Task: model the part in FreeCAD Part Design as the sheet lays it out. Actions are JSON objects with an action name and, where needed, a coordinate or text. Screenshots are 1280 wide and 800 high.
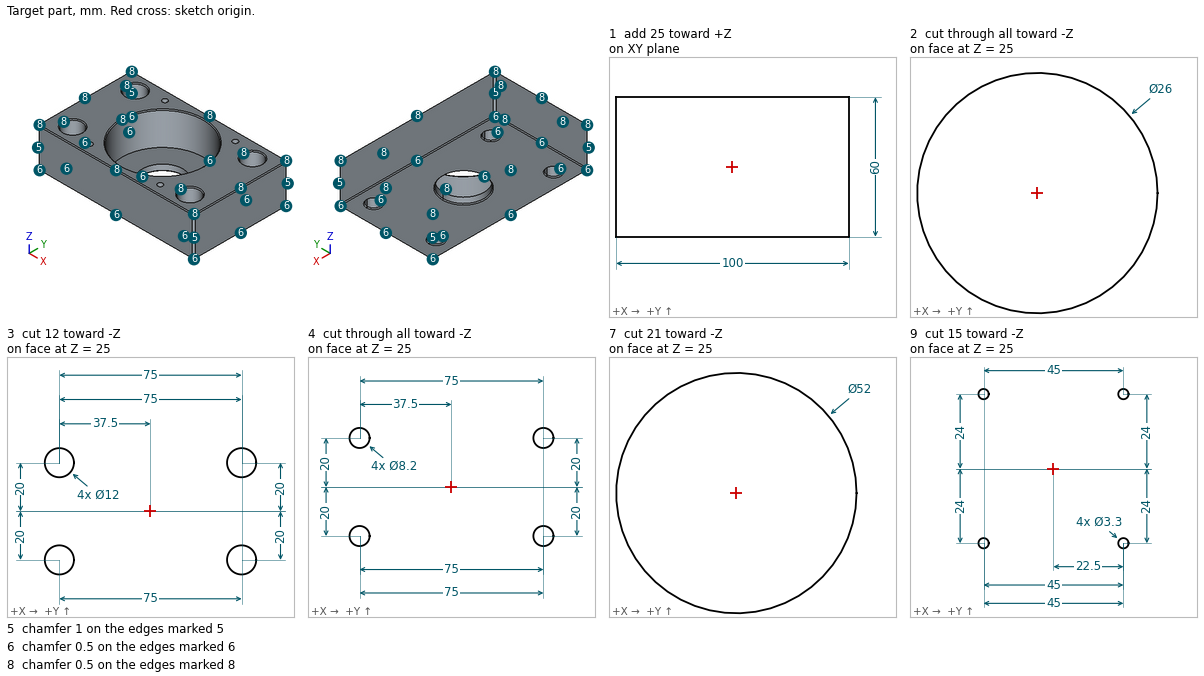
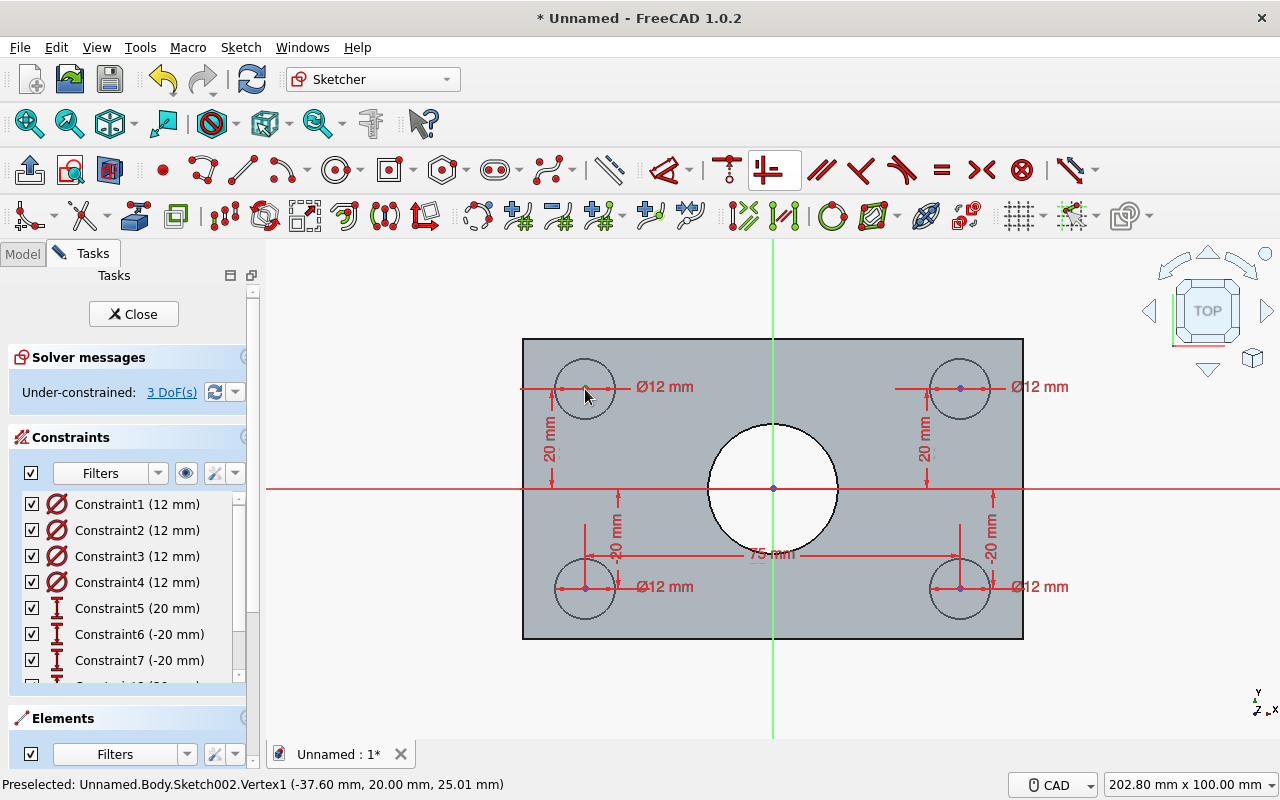
{"action": "left_click", "coordinate": [960, 589]}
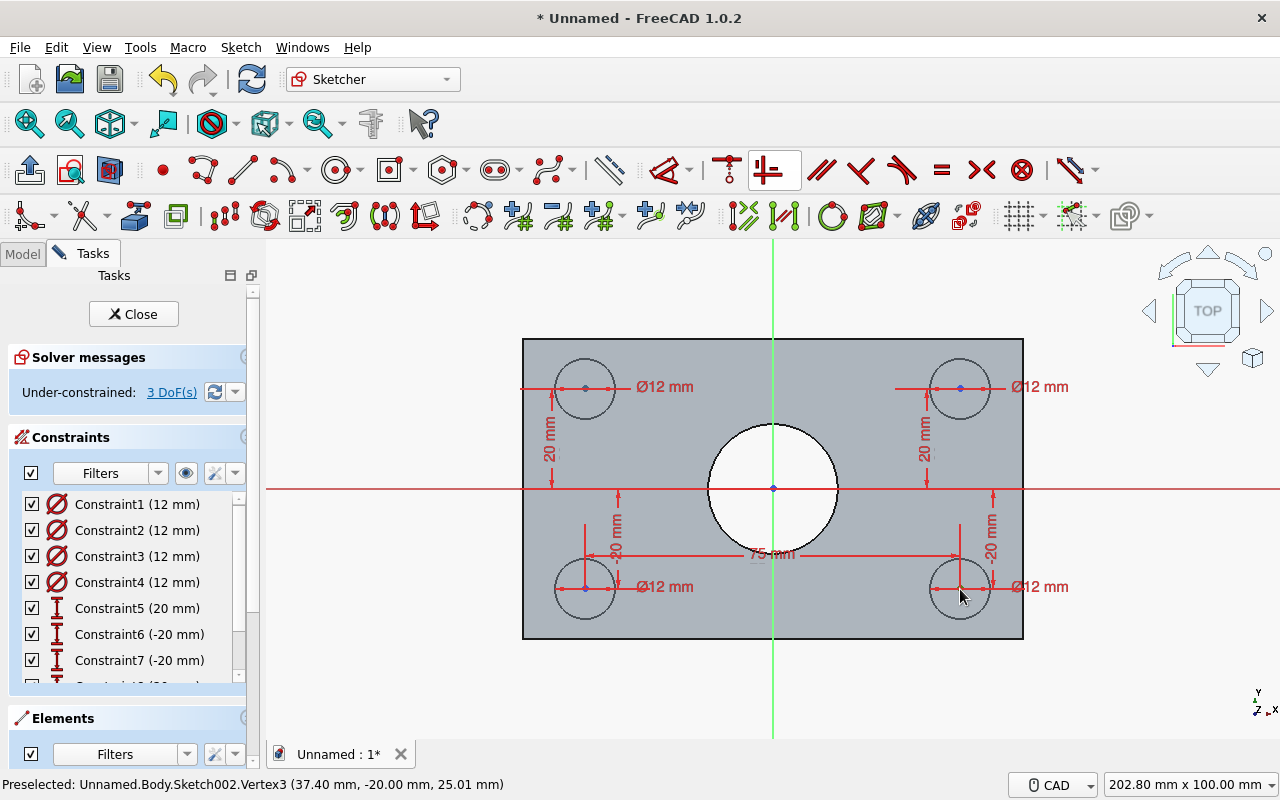
{"action": "key", "text": "l"}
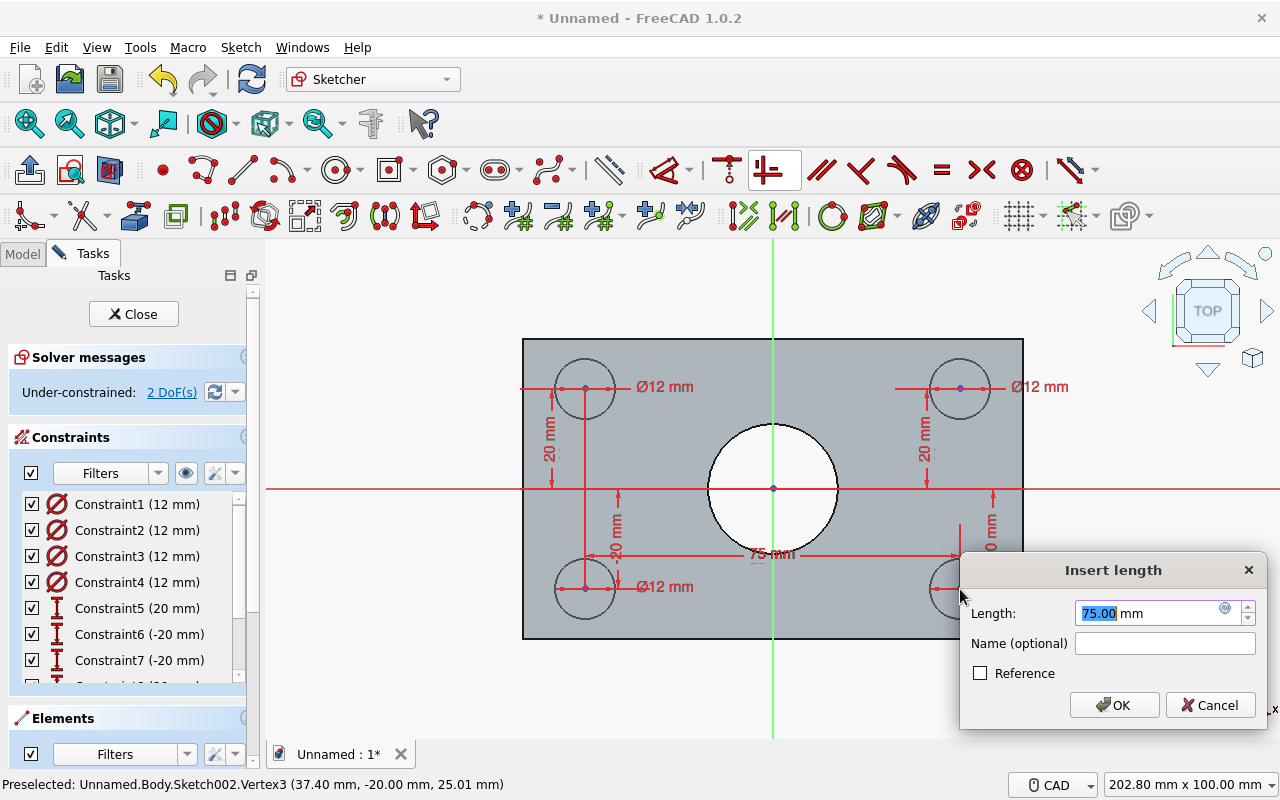
{"action": "type", "text": "75"}
{"action": "key", "text": "Return"}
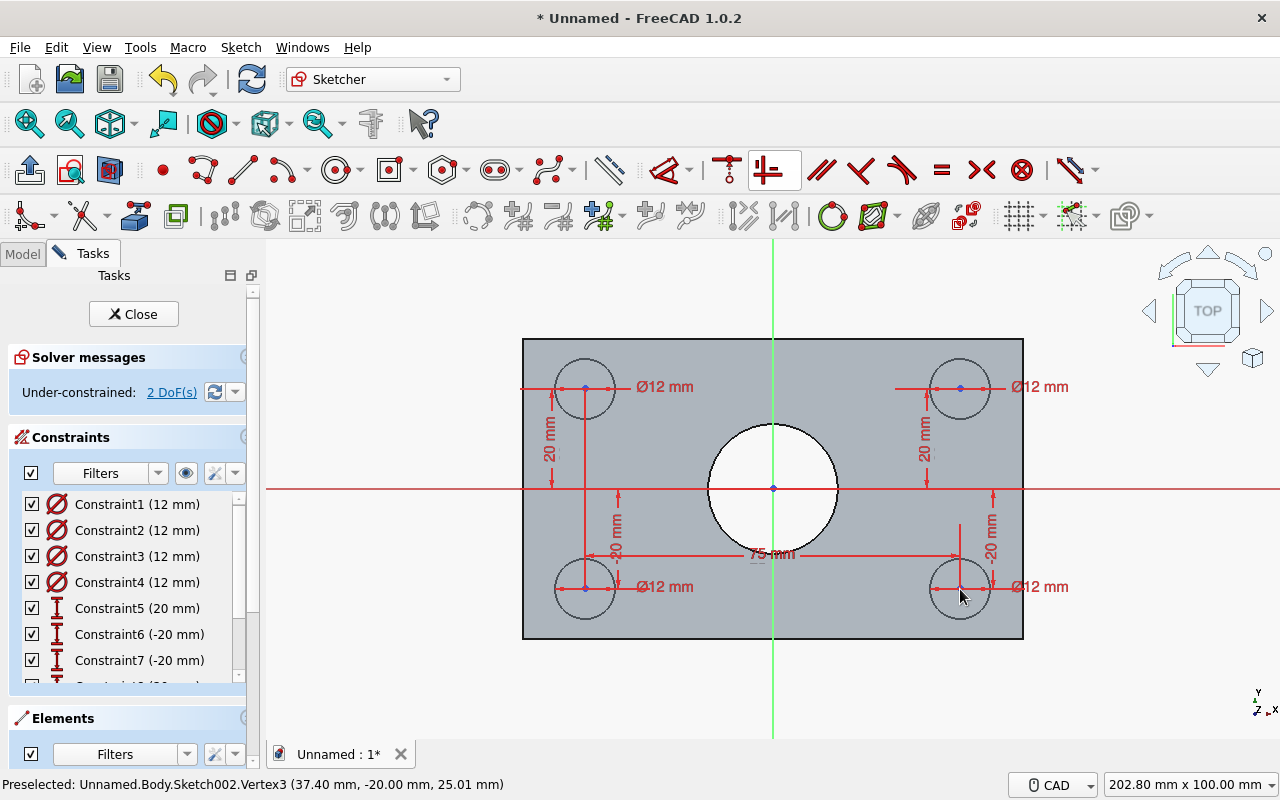
{"action": "left_click", "coordinate": [585, 389]}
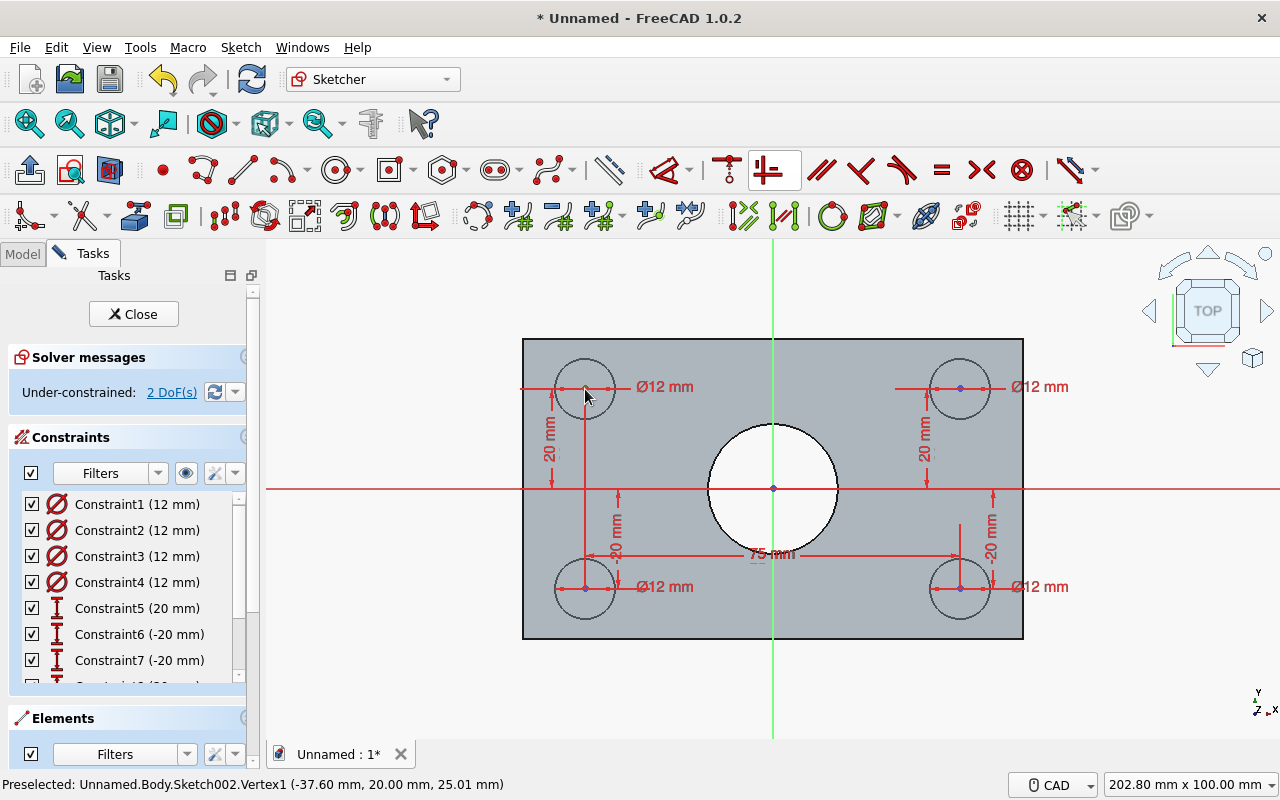
{"action": "left_click", "coordinate": [960, 389]}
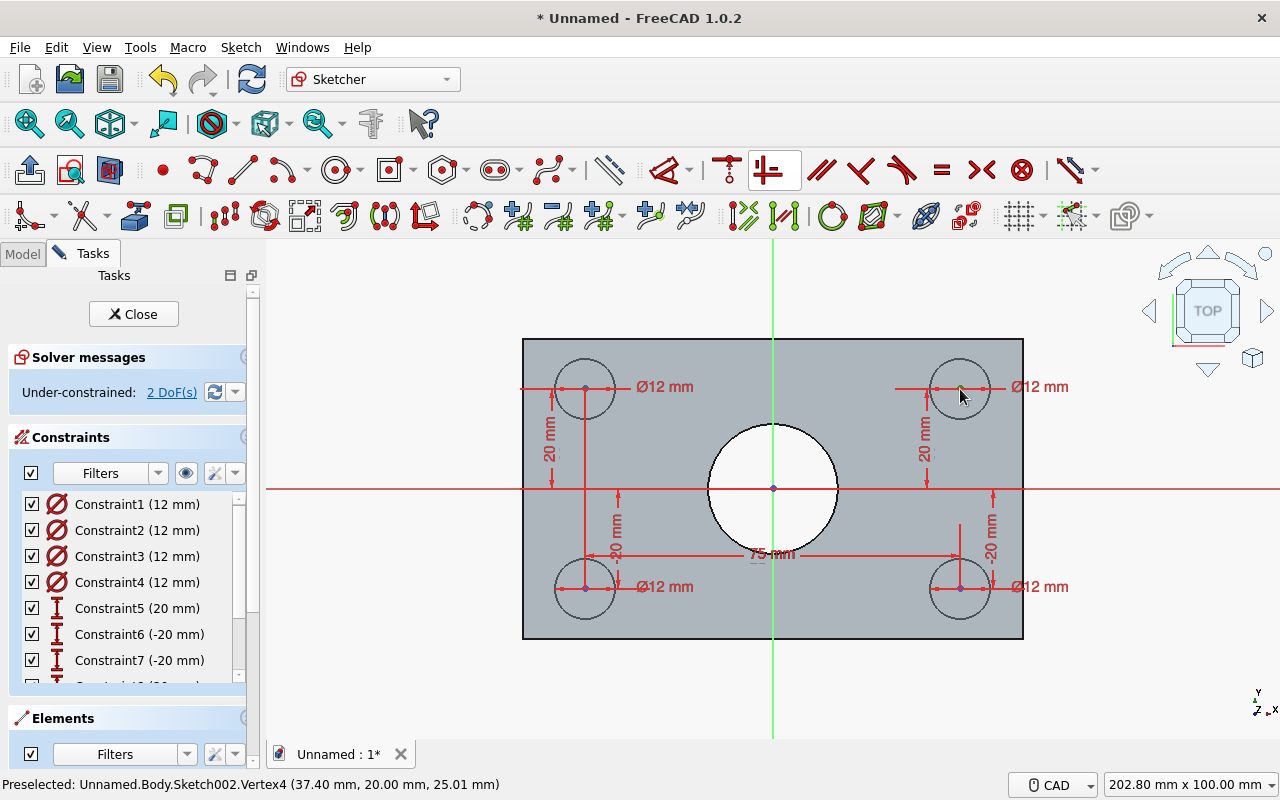
{"action": "key", "text": "l"}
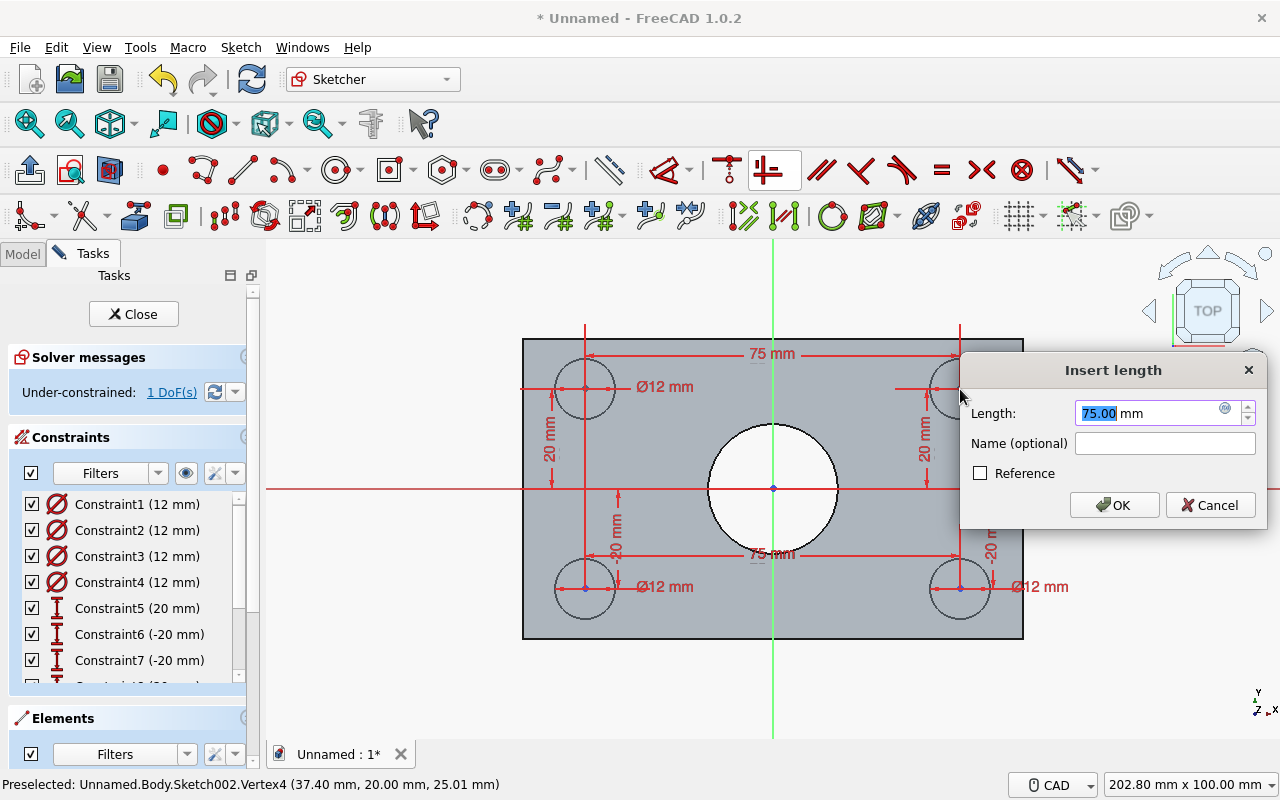
{"action": "type", "text": "75"}
{"action": "key", "text": "Return"}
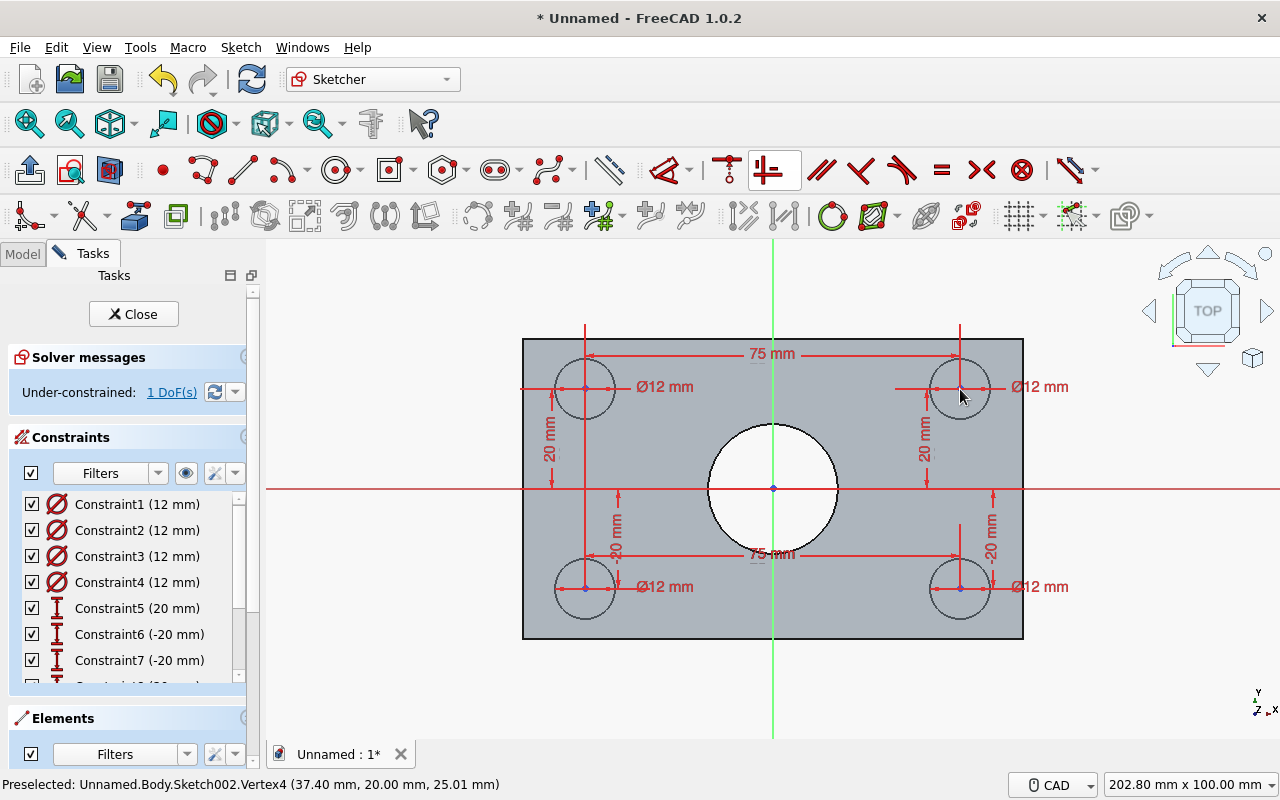
{"action": "left_click", "coordinate": [585, 389]}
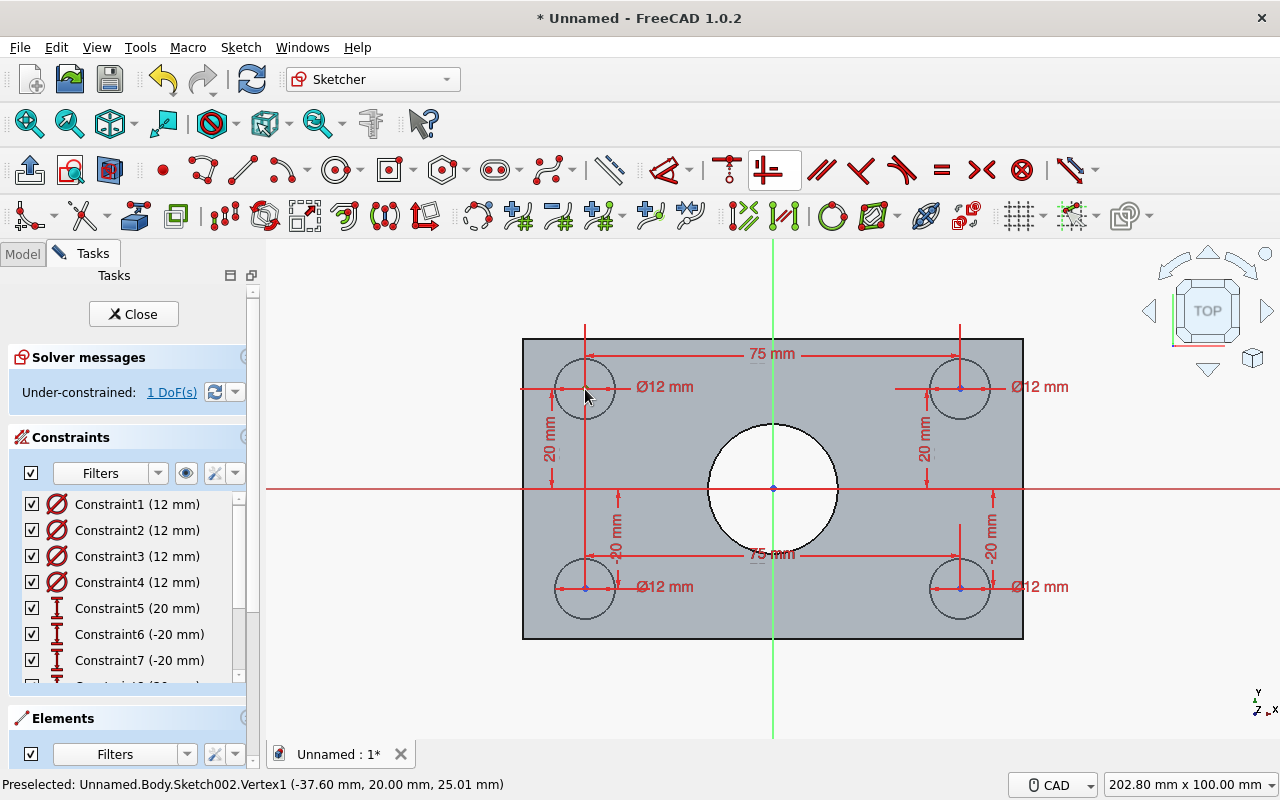
{"action": "key", "text": "l"}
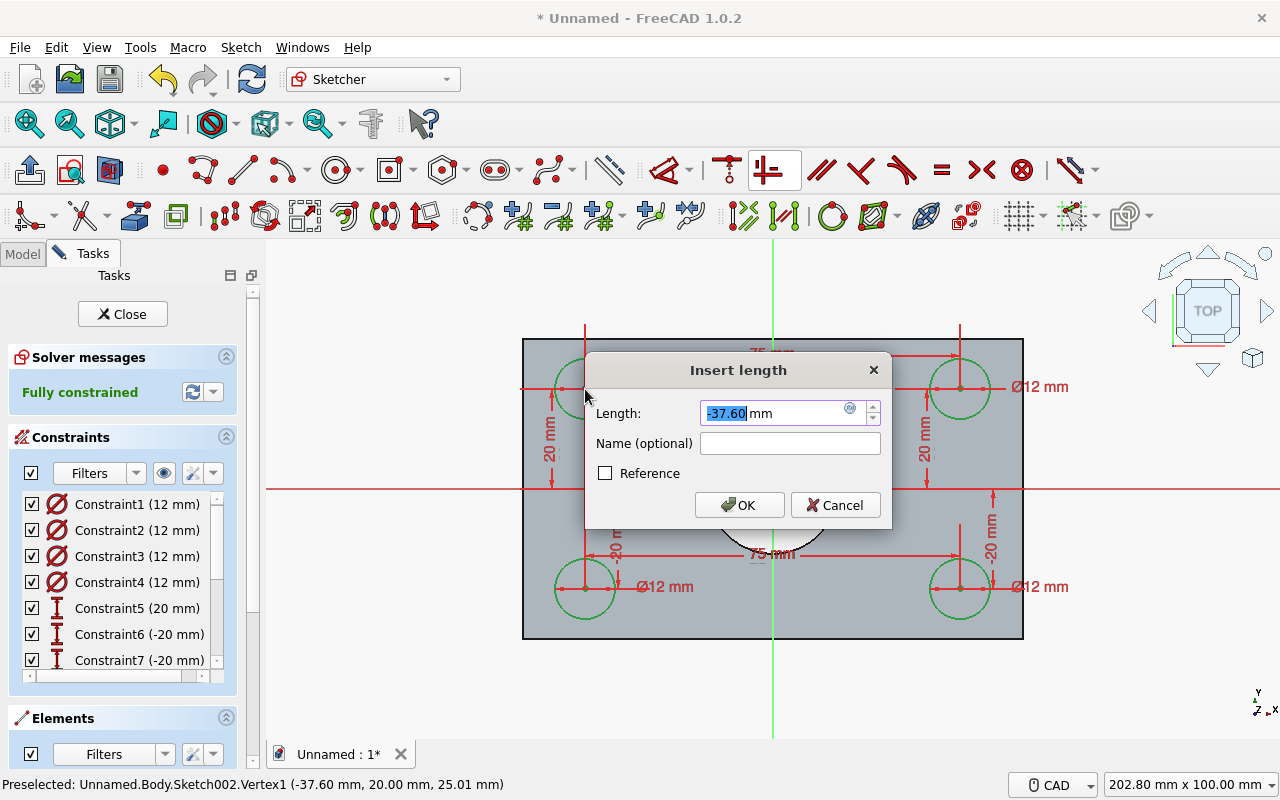
{"action": "type", "text": "-37.5"}
{"action": "key", "text": "Return"}